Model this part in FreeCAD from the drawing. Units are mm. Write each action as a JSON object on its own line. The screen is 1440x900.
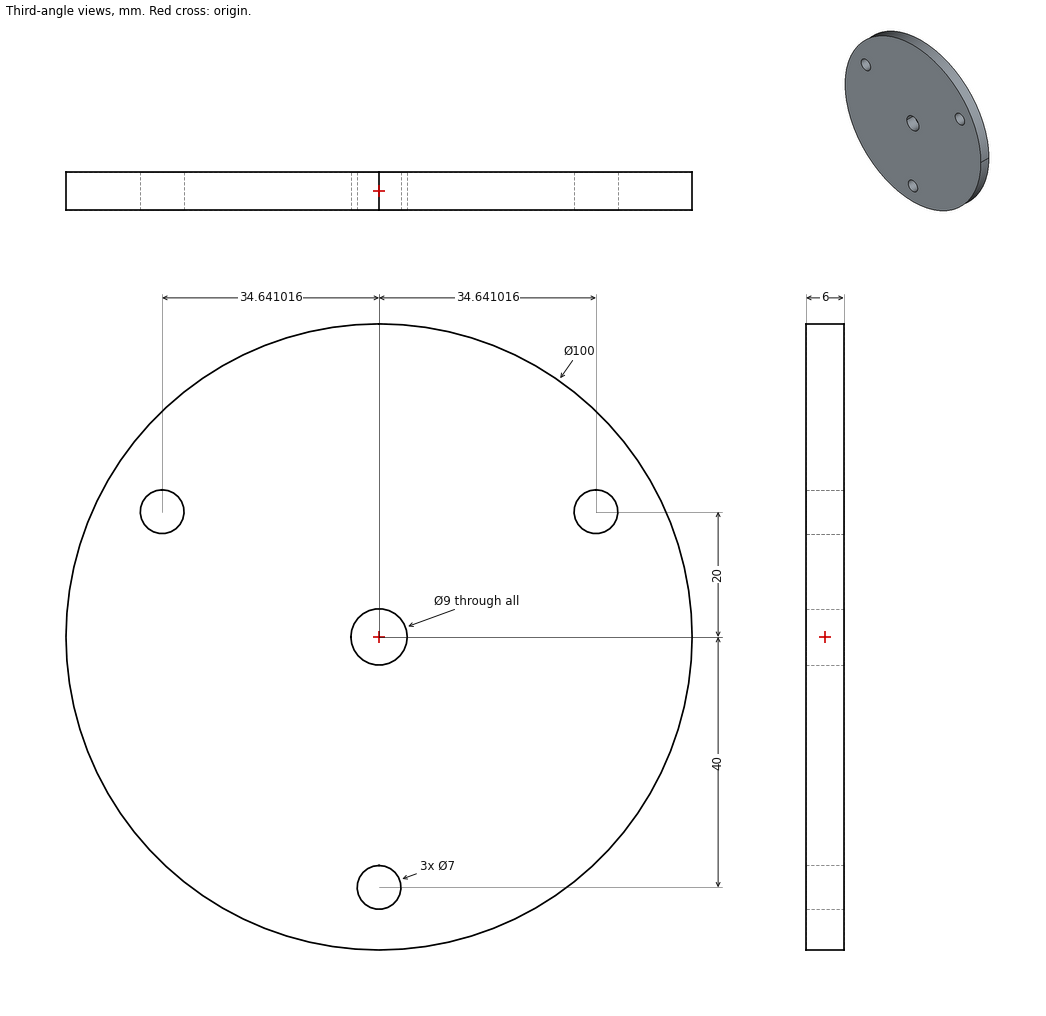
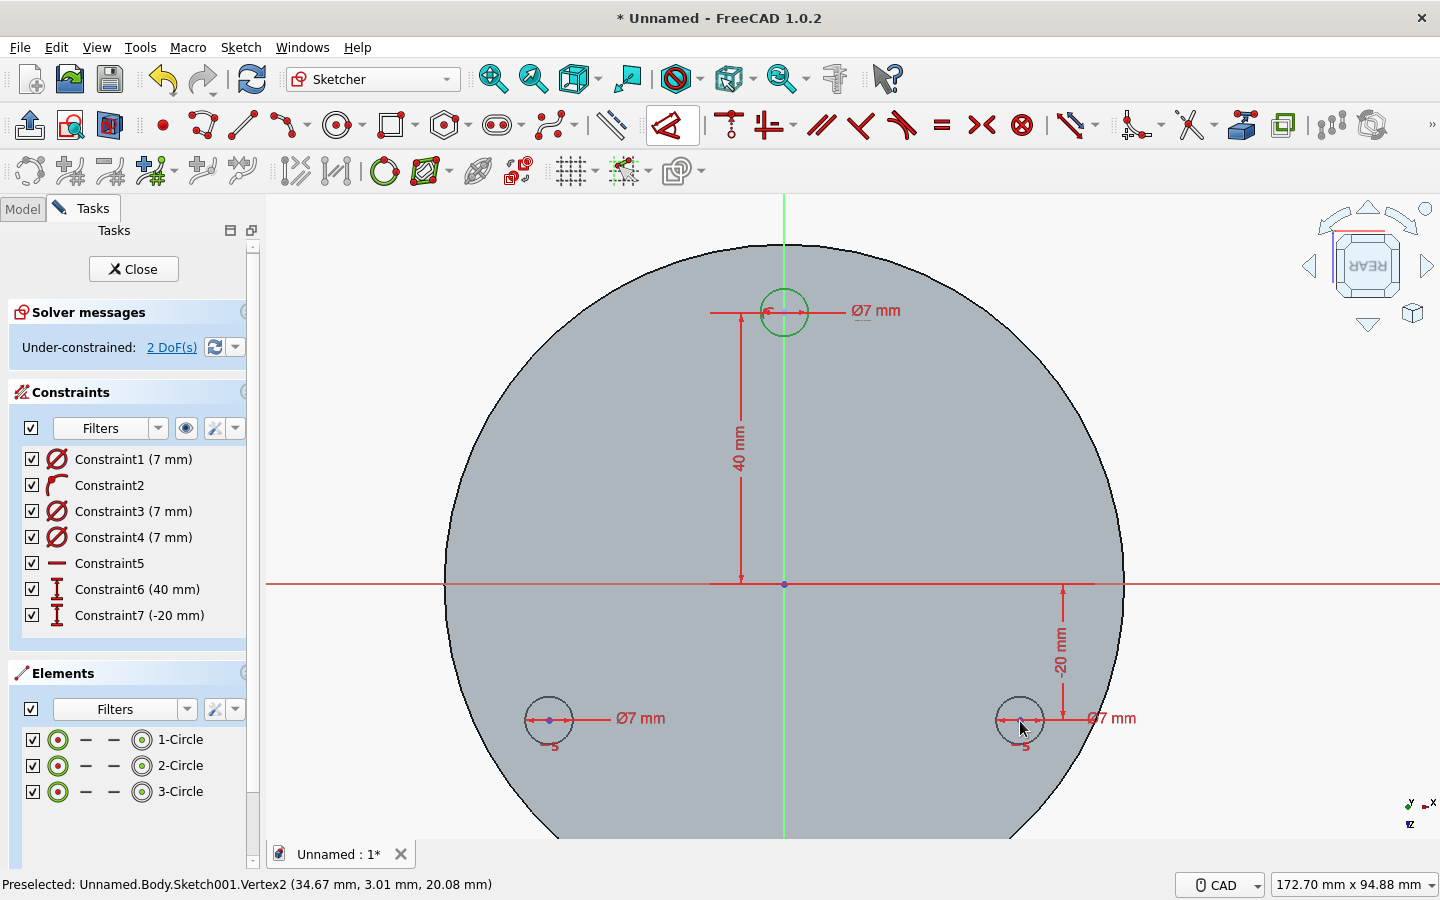
{"action": "left_click", "coordinate": [1020, 720]}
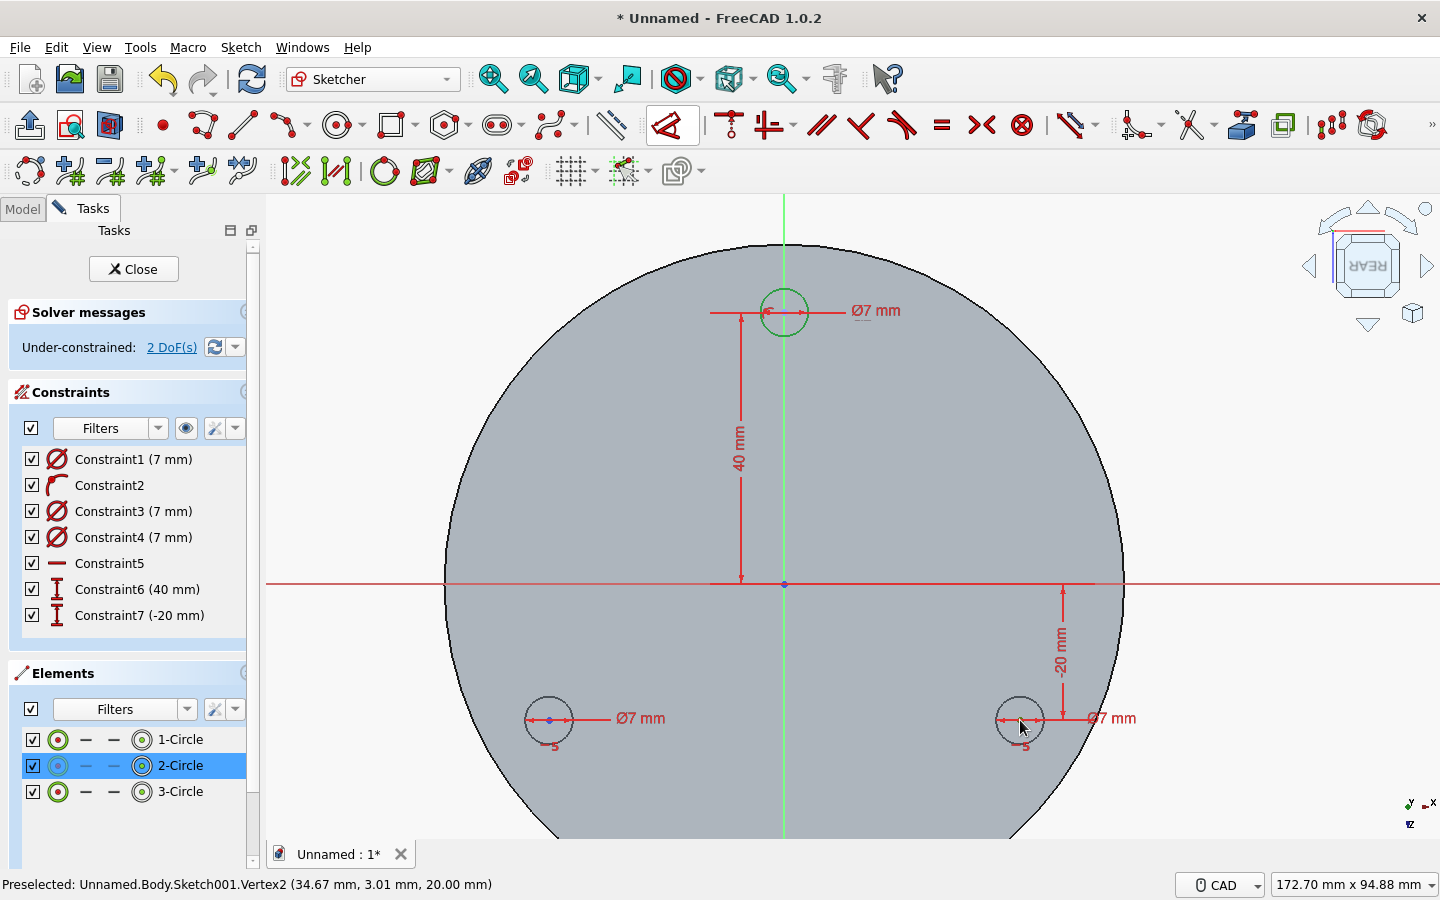
{"action": "left_click", "coordinate": [694, 126]}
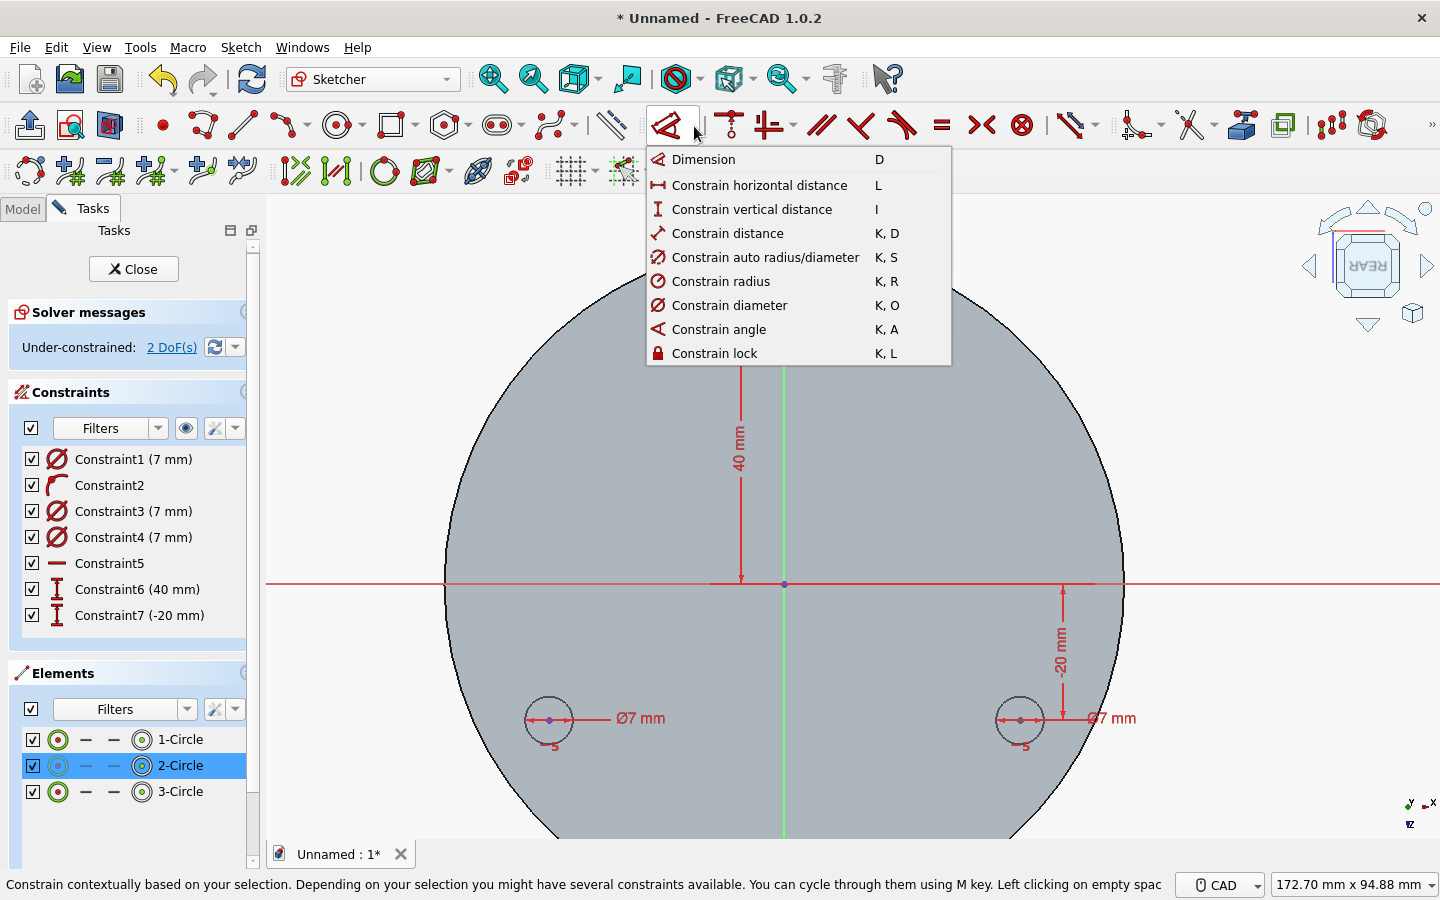
{"action": "left_click", "coordinate": [799, 185]}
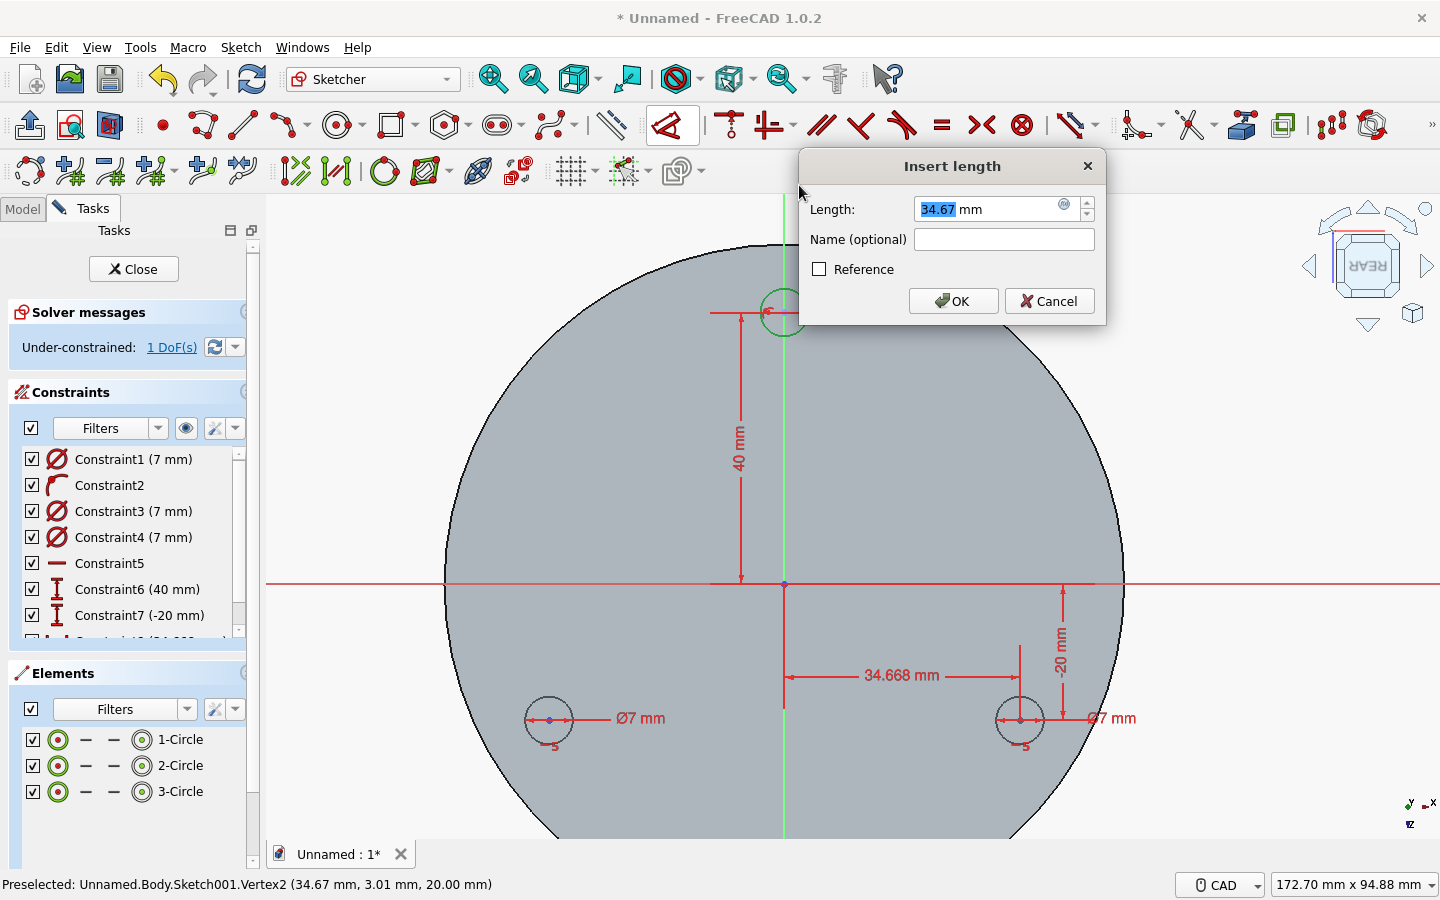
{"action": "type", "text": "34.641016"}
{"action": "key", "text": "Return"}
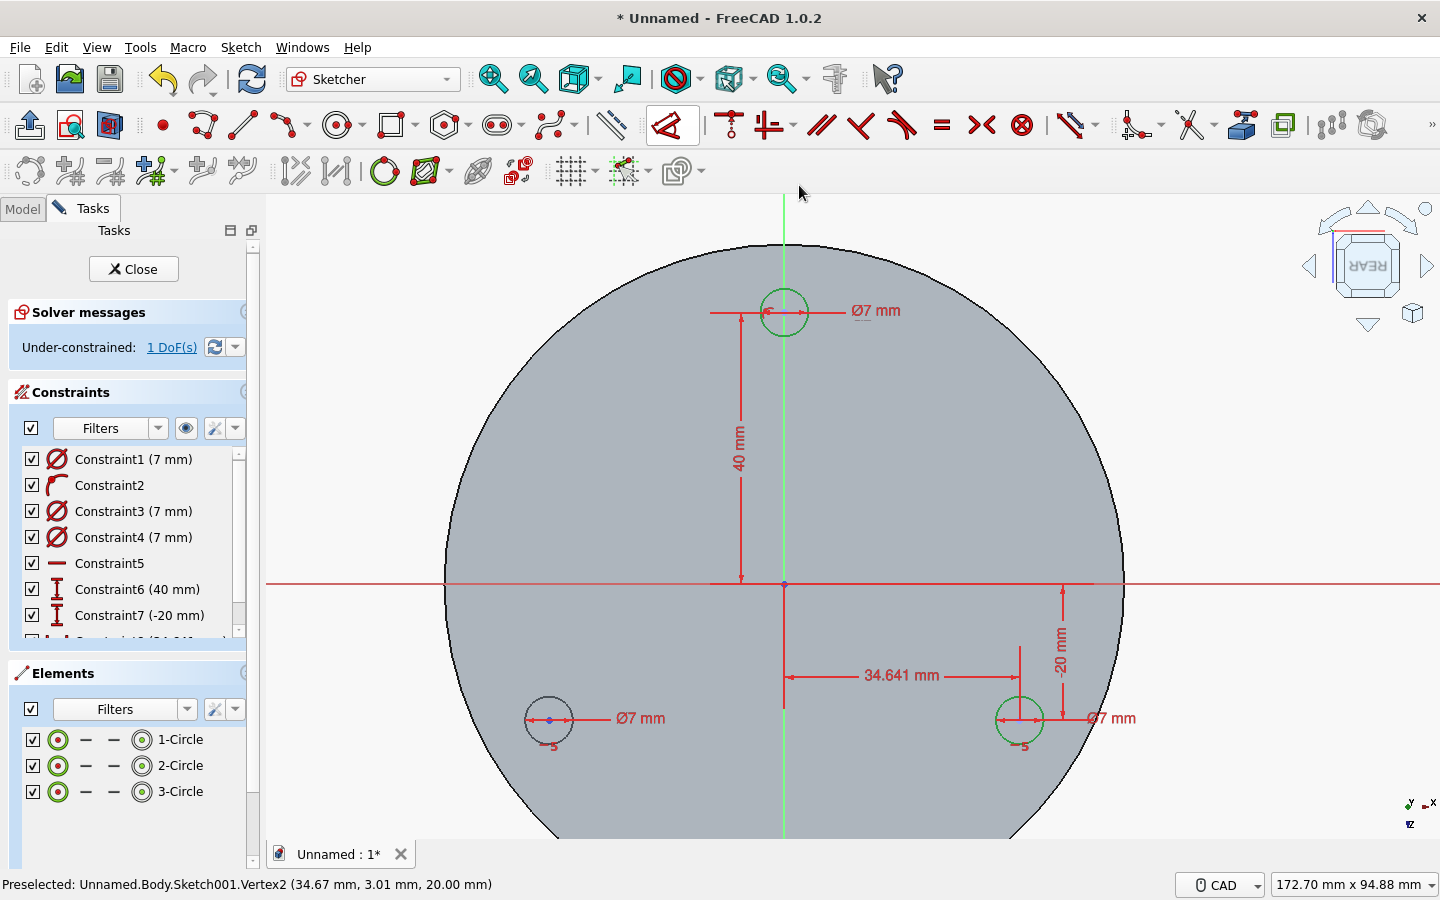
{"action": "left_click", "coordinate": [549, 720]}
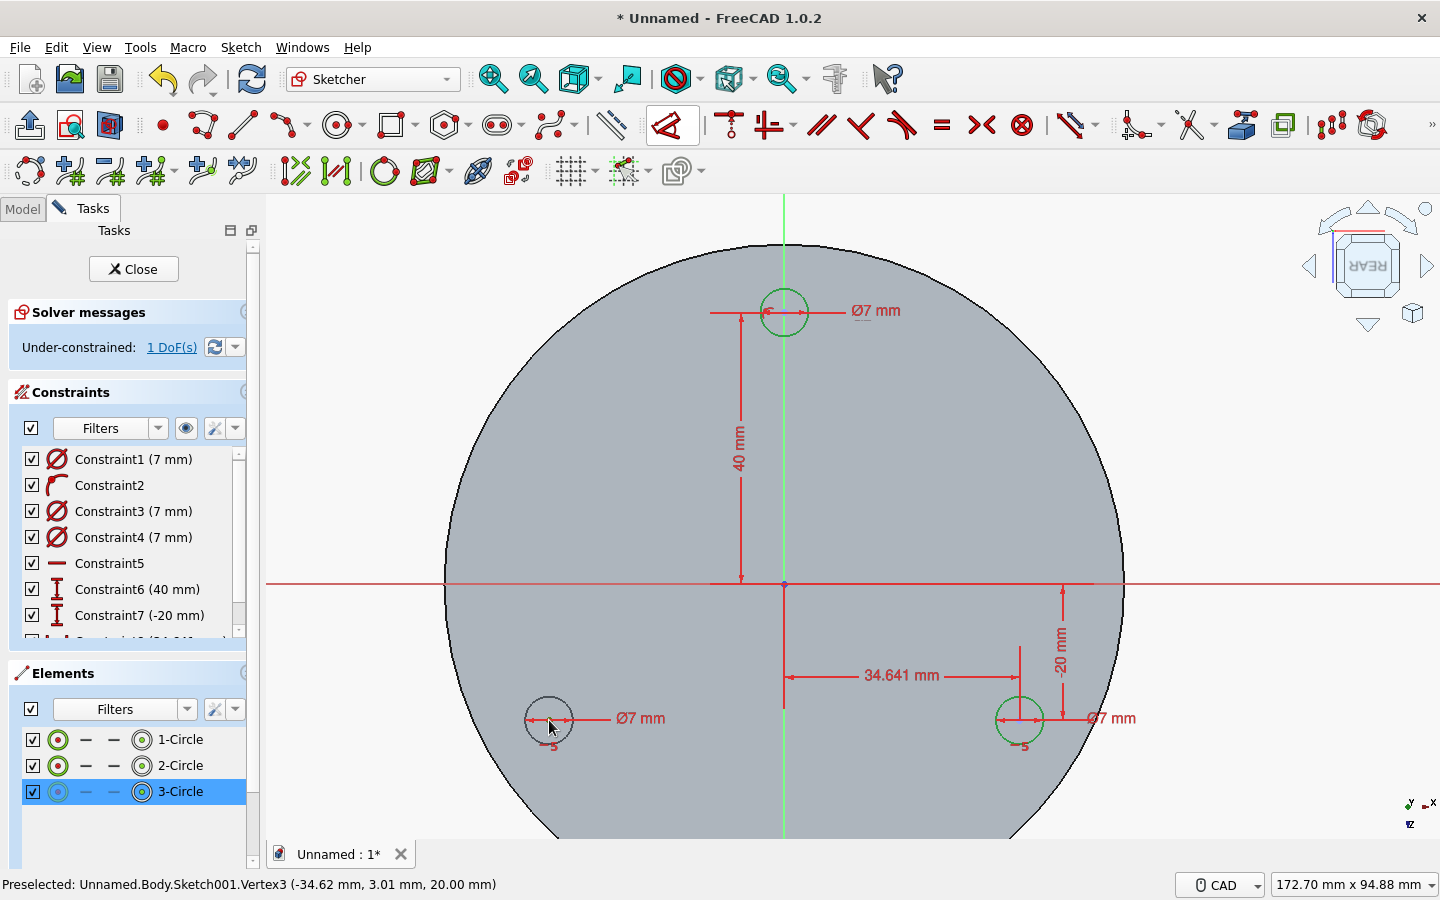
{"action": "key", "text": "l"}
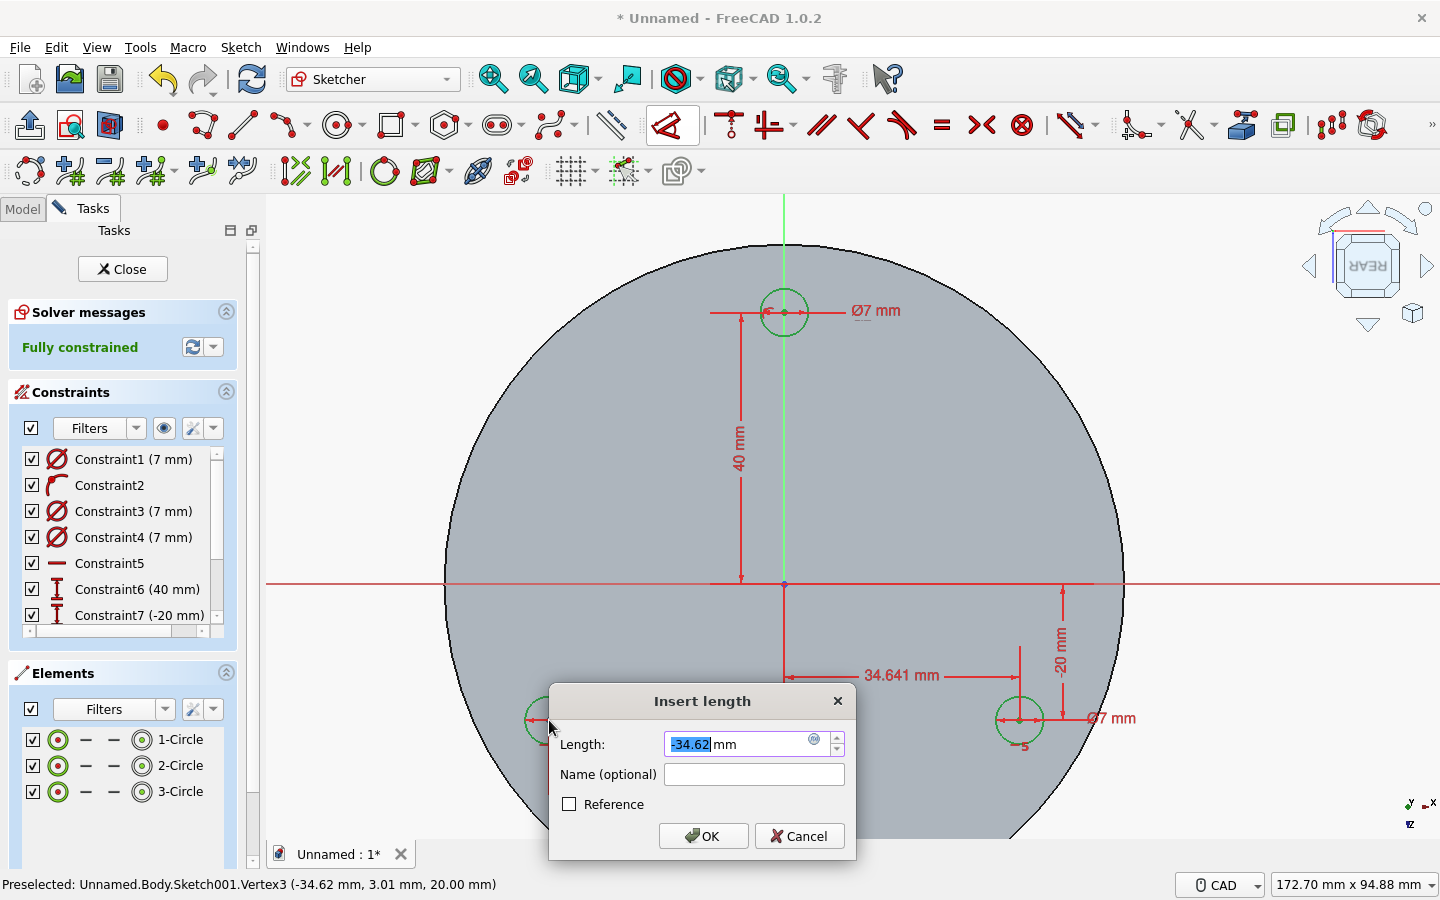
{"action": "type", "text": "-34.641016"}
{"action": "key", "text": "Return"}